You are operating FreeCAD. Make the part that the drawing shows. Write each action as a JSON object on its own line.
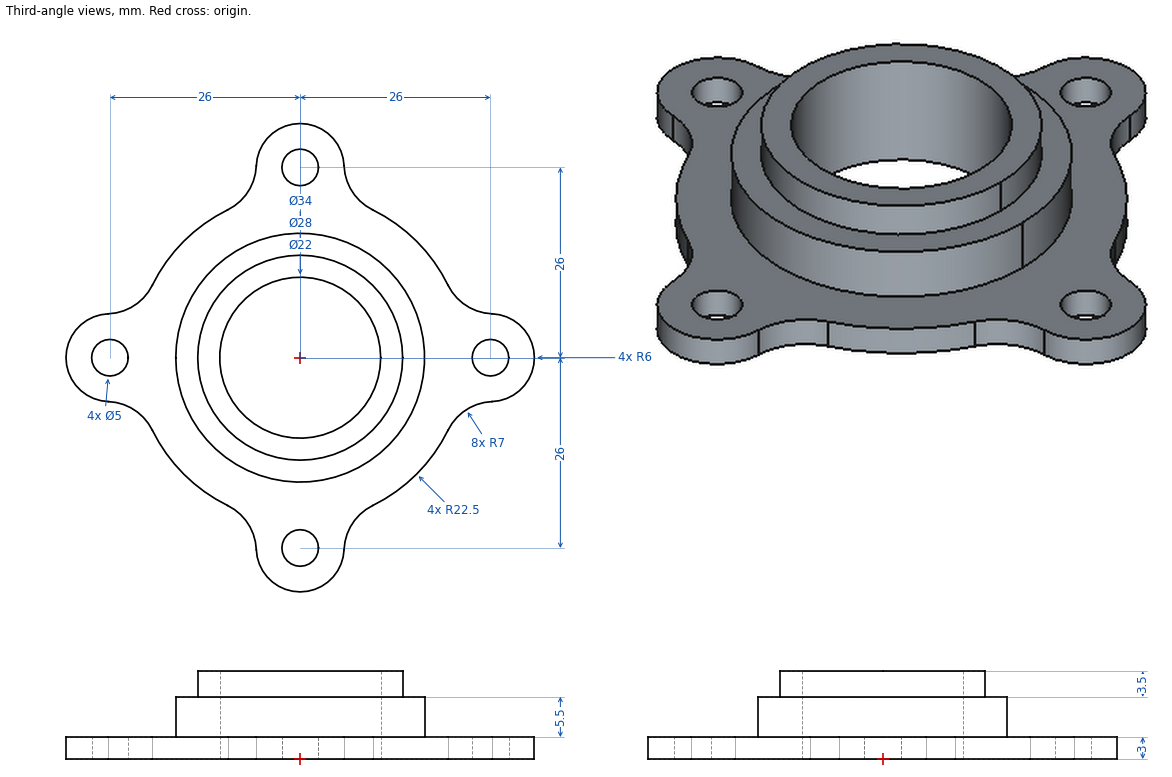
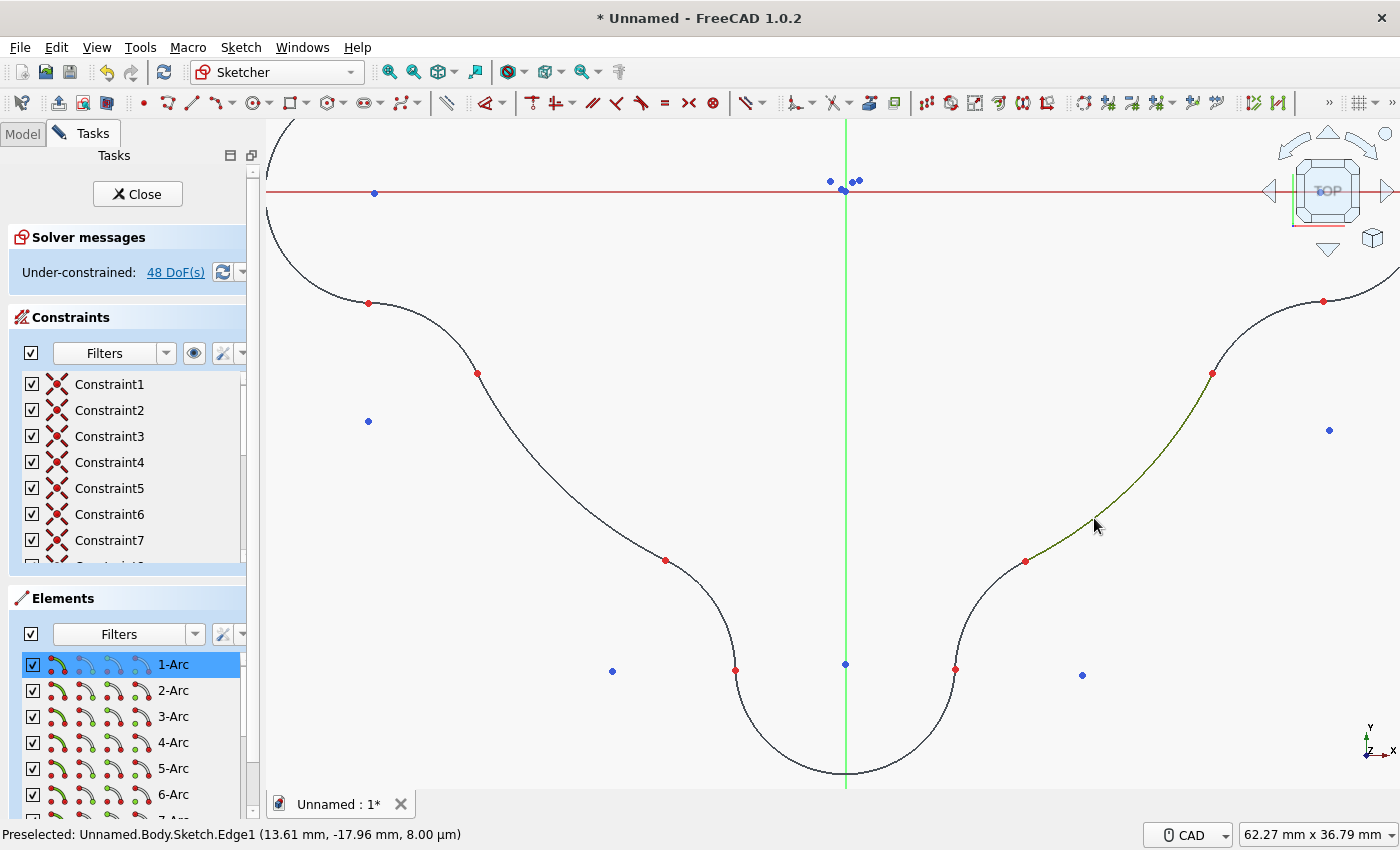
{"action": "left_click", "coordinate": [1228, 350]}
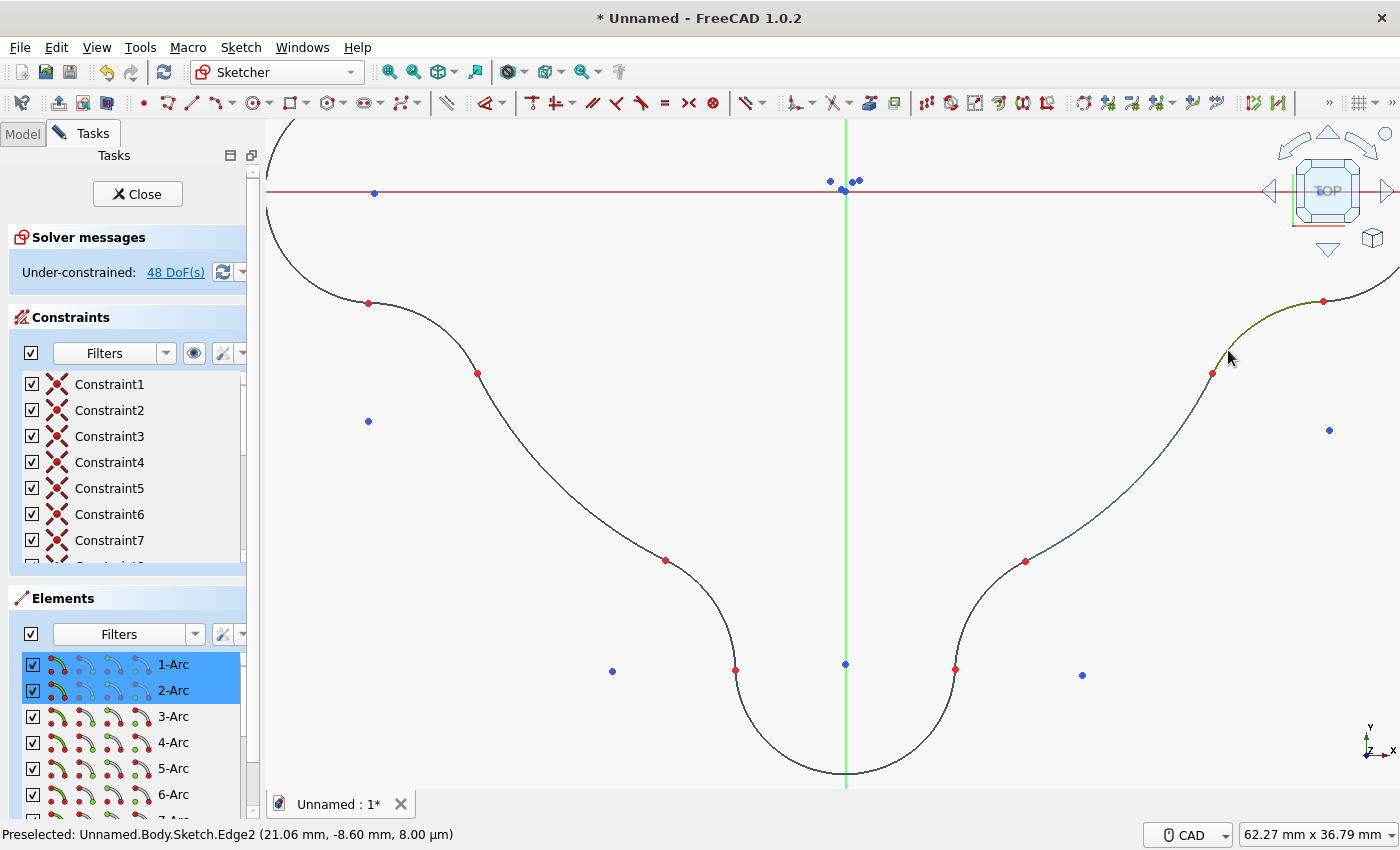
{"action": "left_click", "coordinate": [642, 104]}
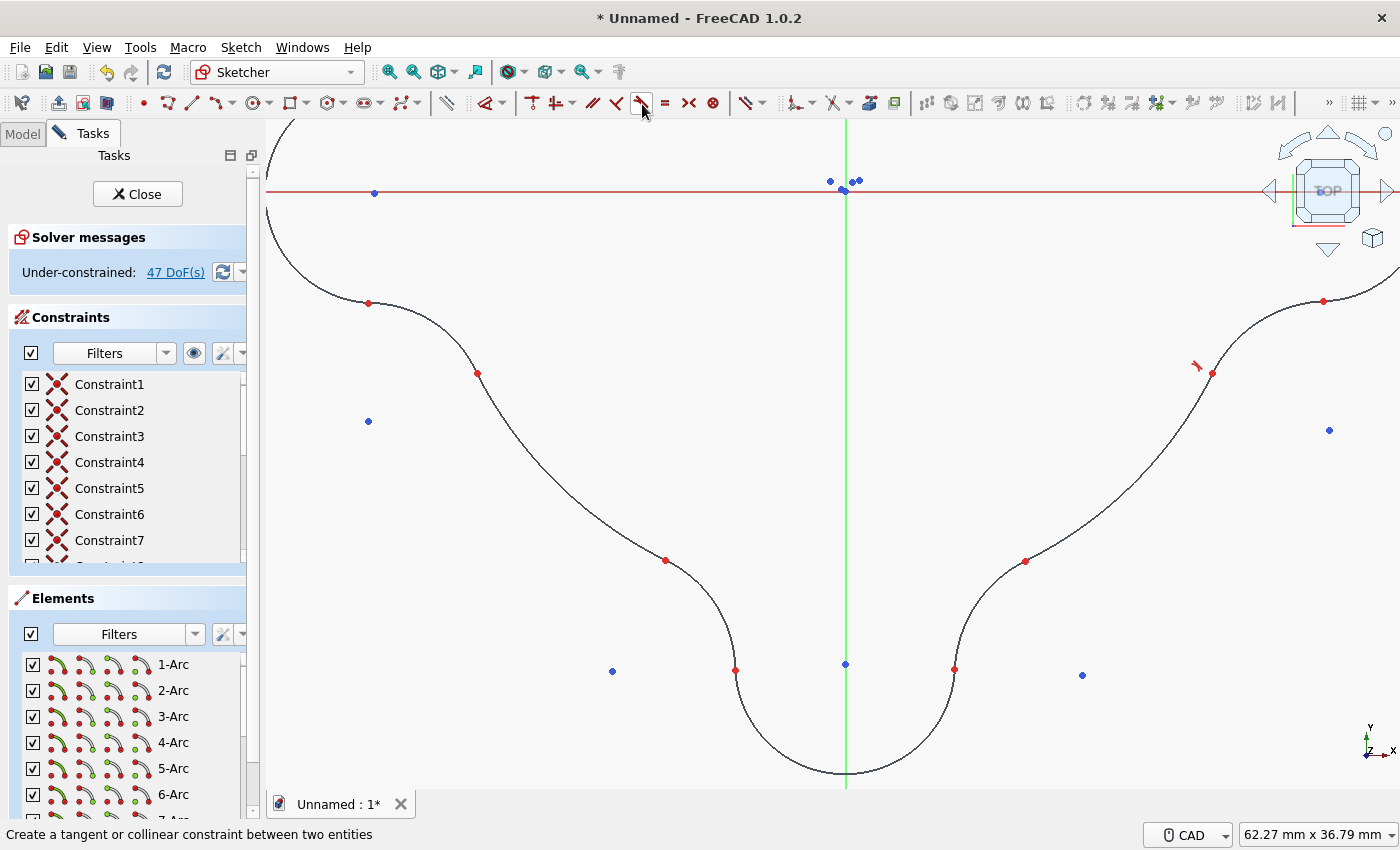
{"action": "left_click", "coordinate": [1094, 518]}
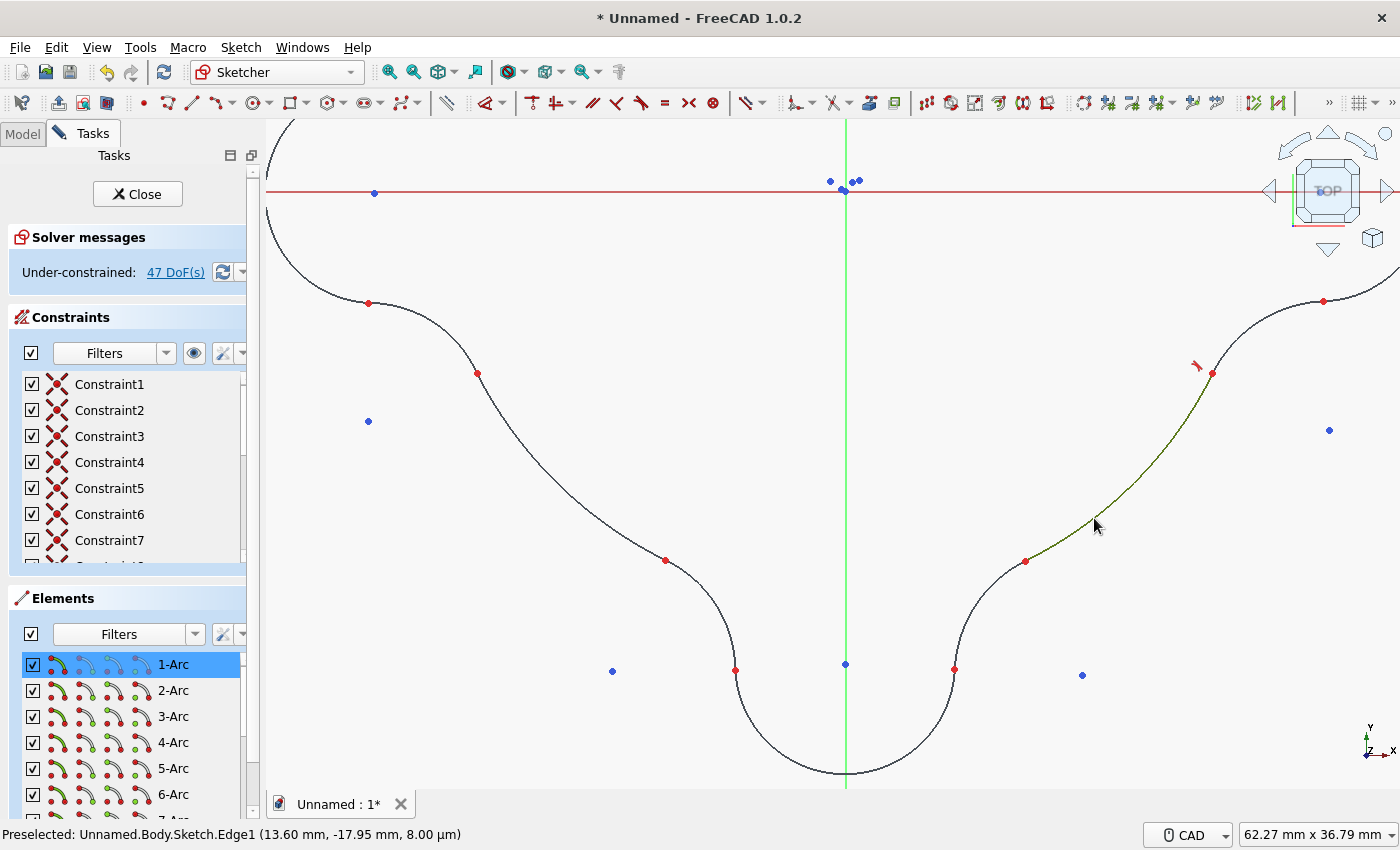
{"action": "left_click", "coordinate": [992, 585]}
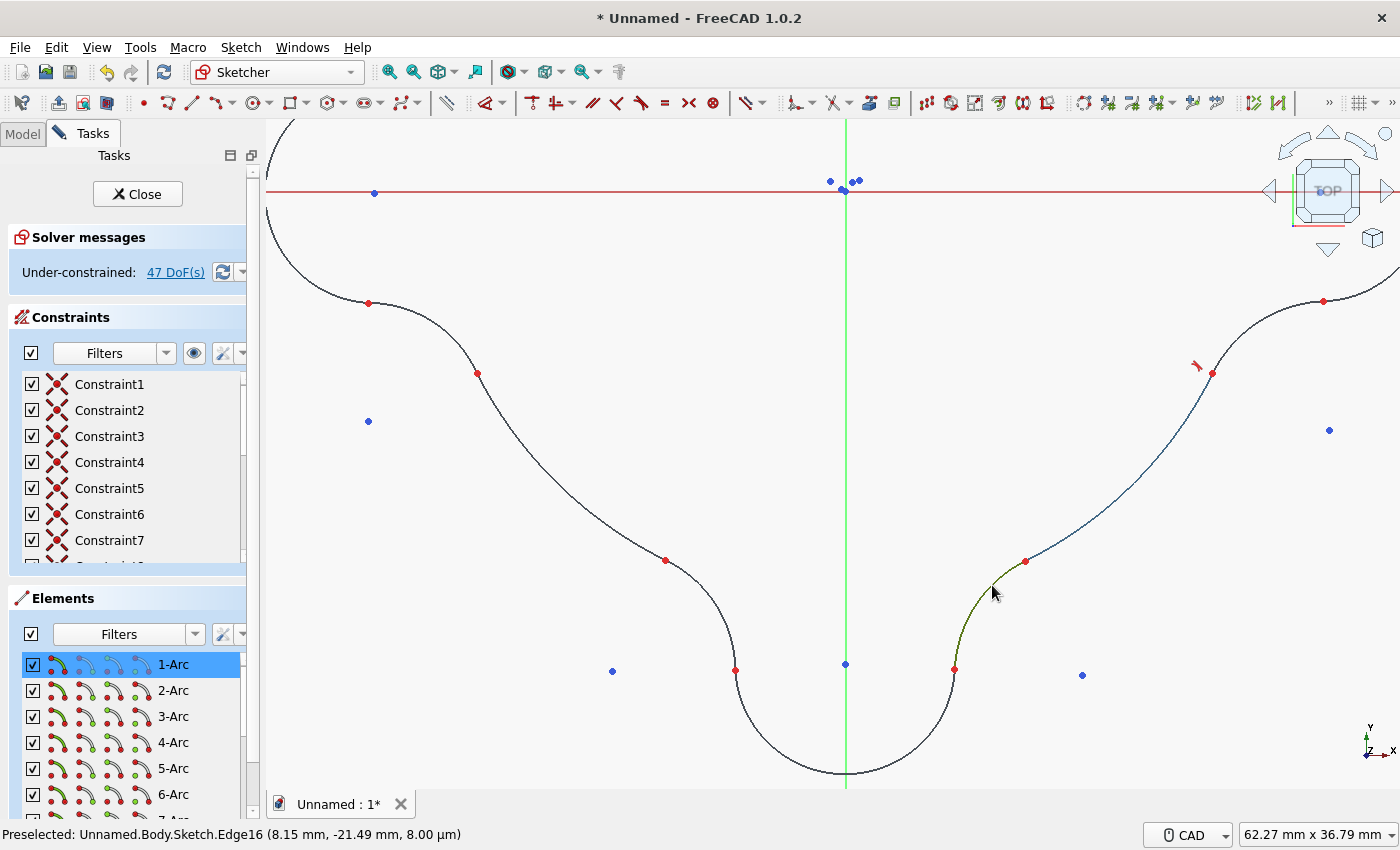
{"action": "left_click", "coordinate": [642, 104]}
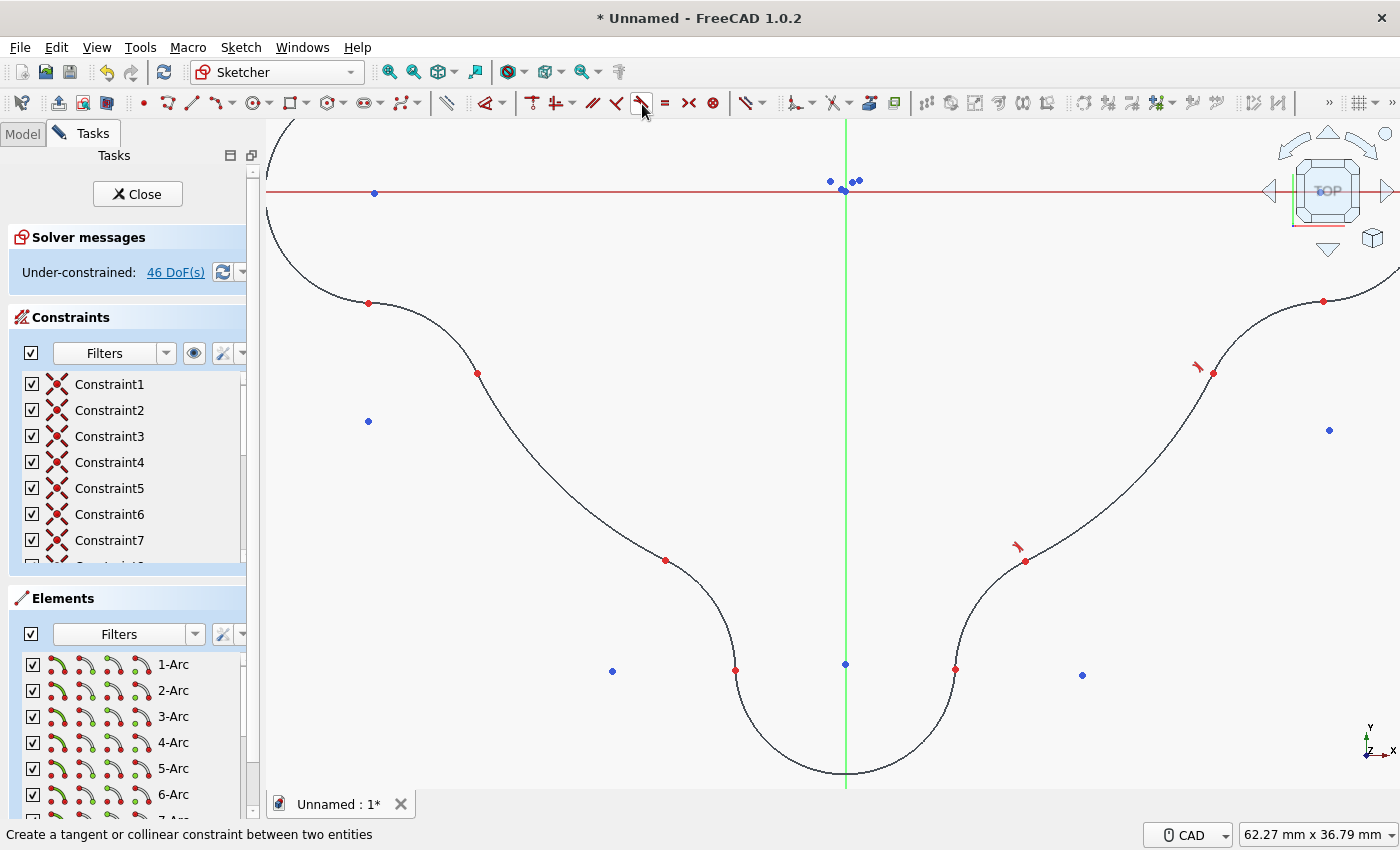
{"action": "left_click", "coordinate": [1228, 350]}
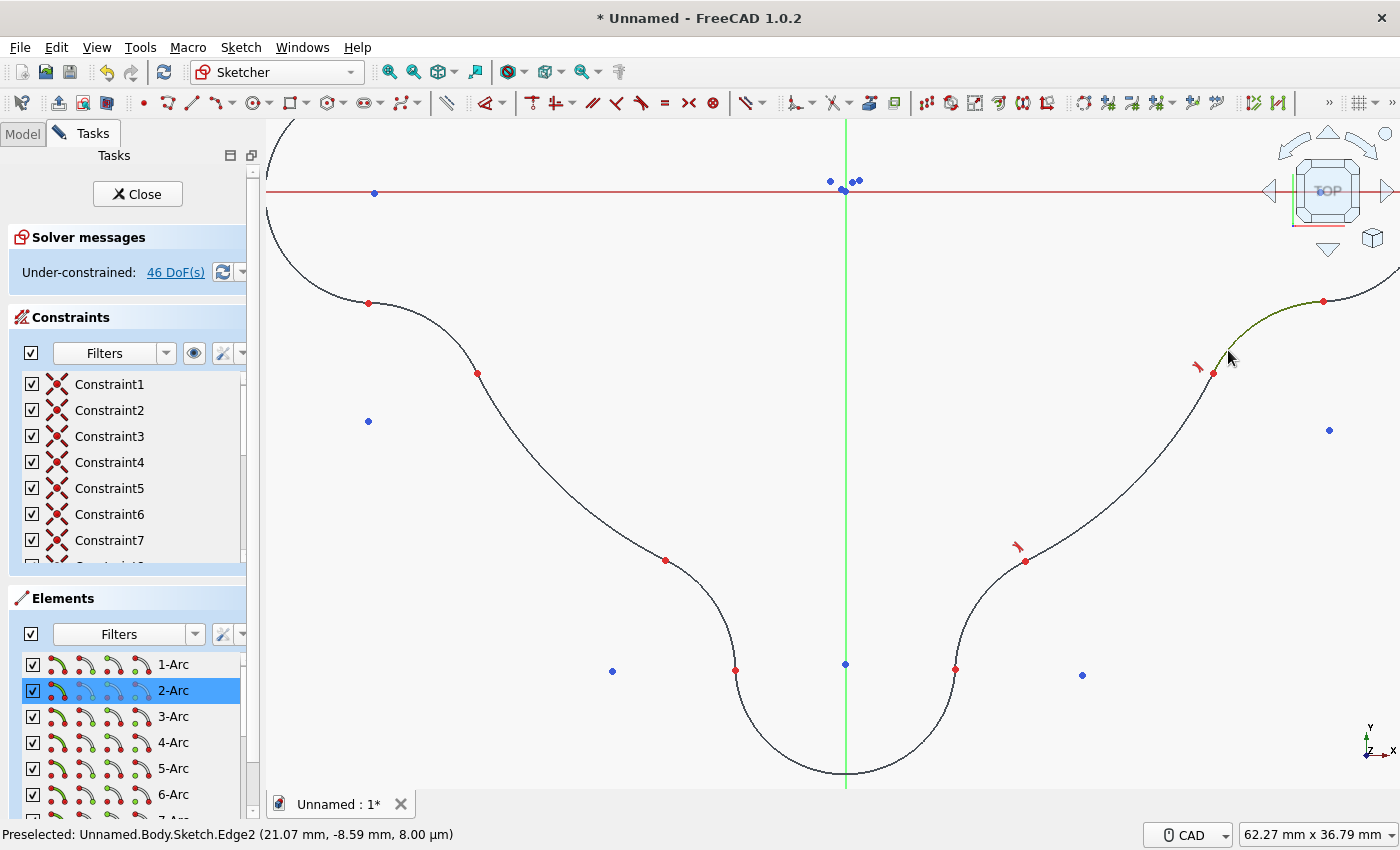
{"action": "scroll", "coordinate": [717, 607], "scroll_direction": "down", "scroll_amount": 5}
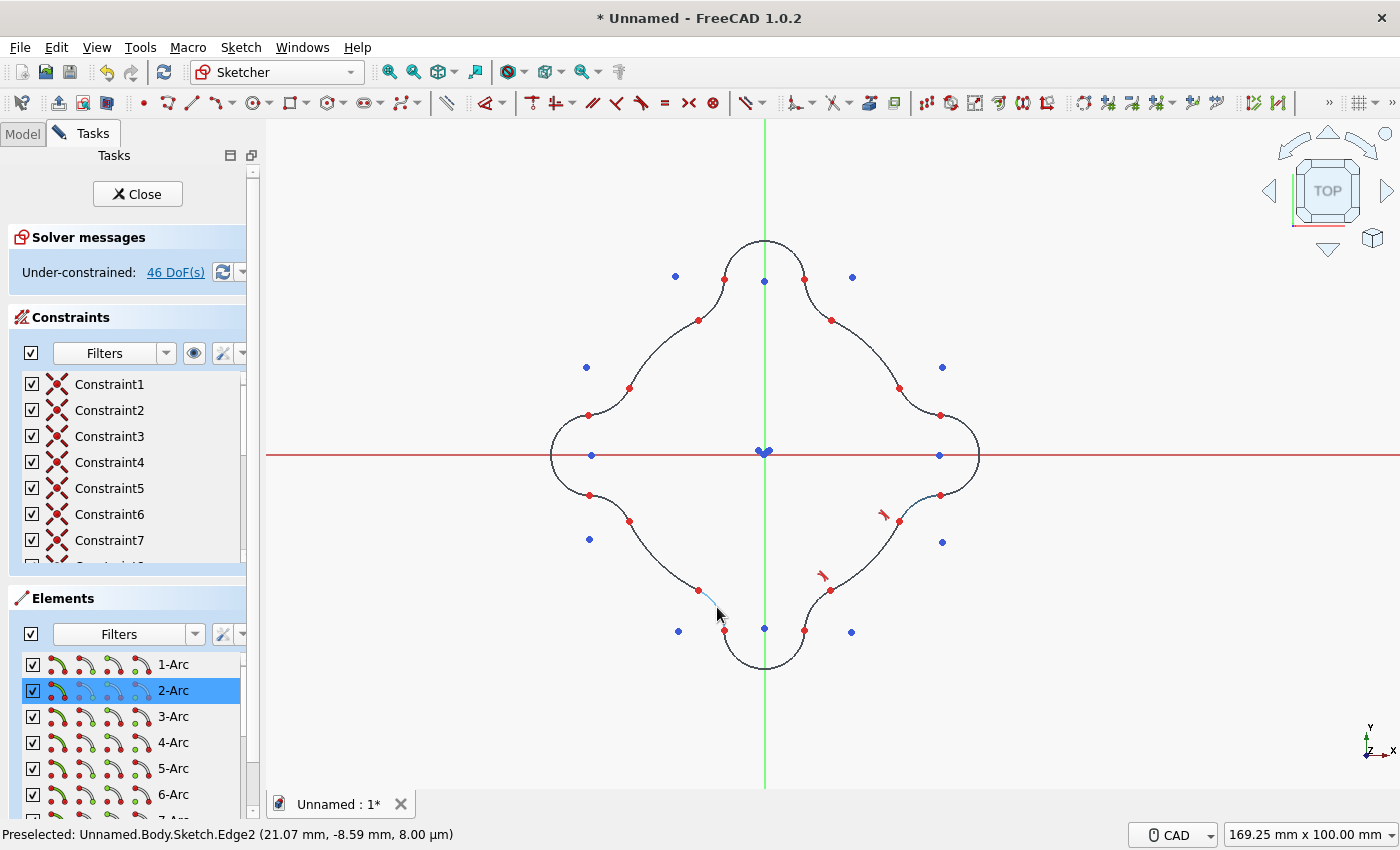
{"action": "left_click", "coordinate": [972, 478]}